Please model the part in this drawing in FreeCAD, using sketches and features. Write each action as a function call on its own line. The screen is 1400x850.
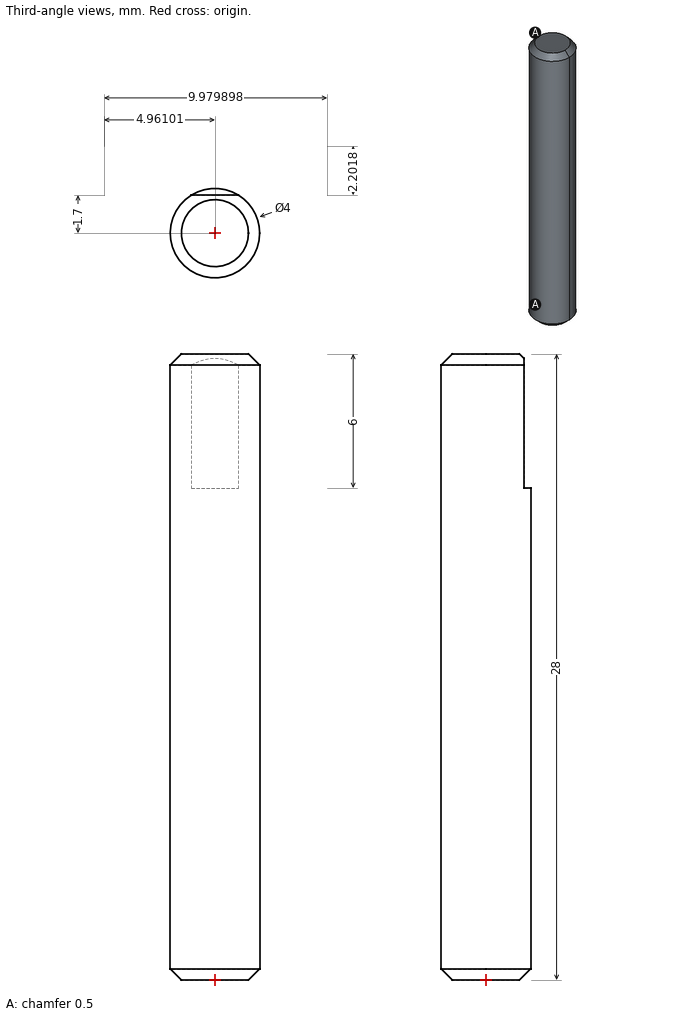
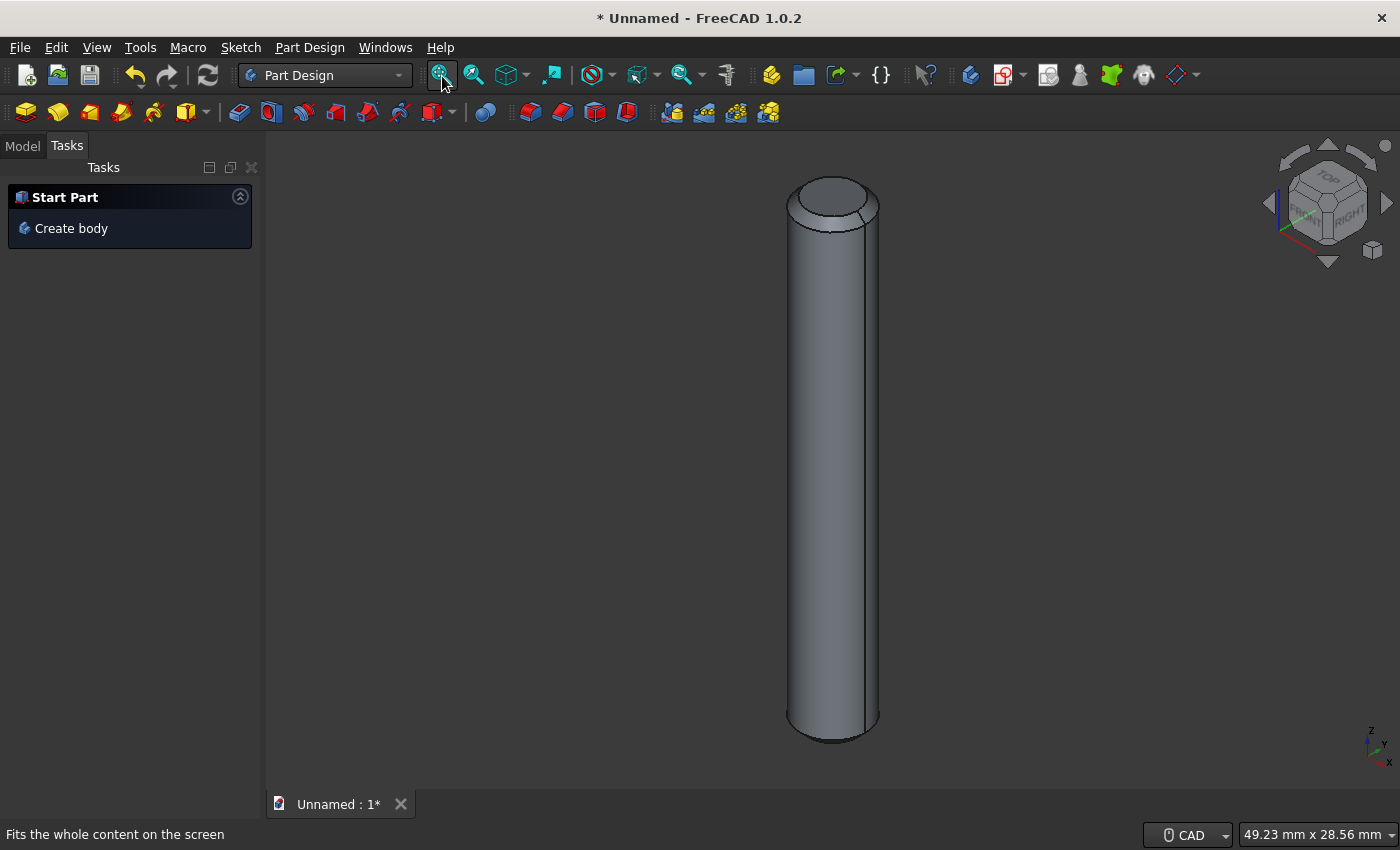
click(833, 196)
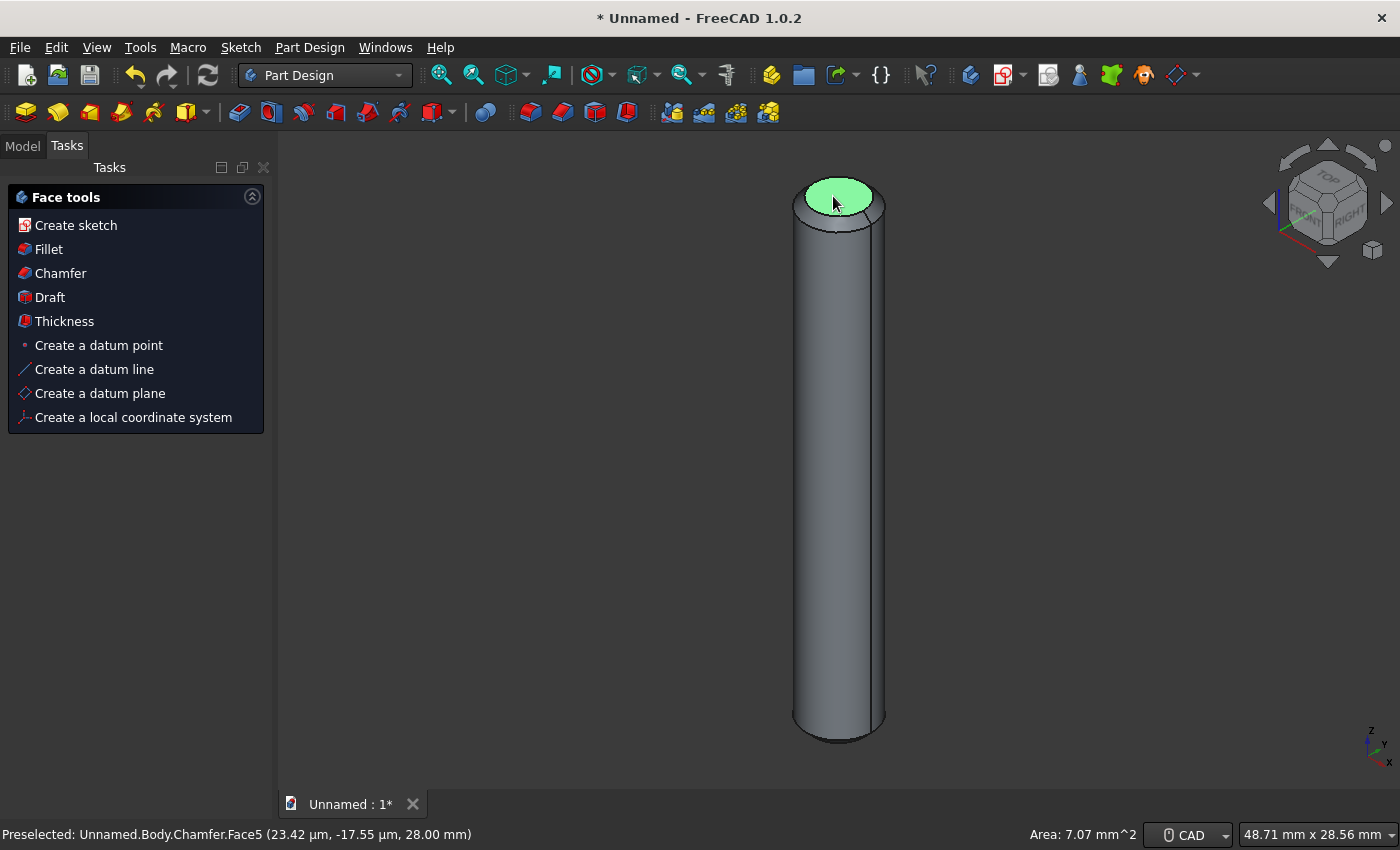
click(1004, 76)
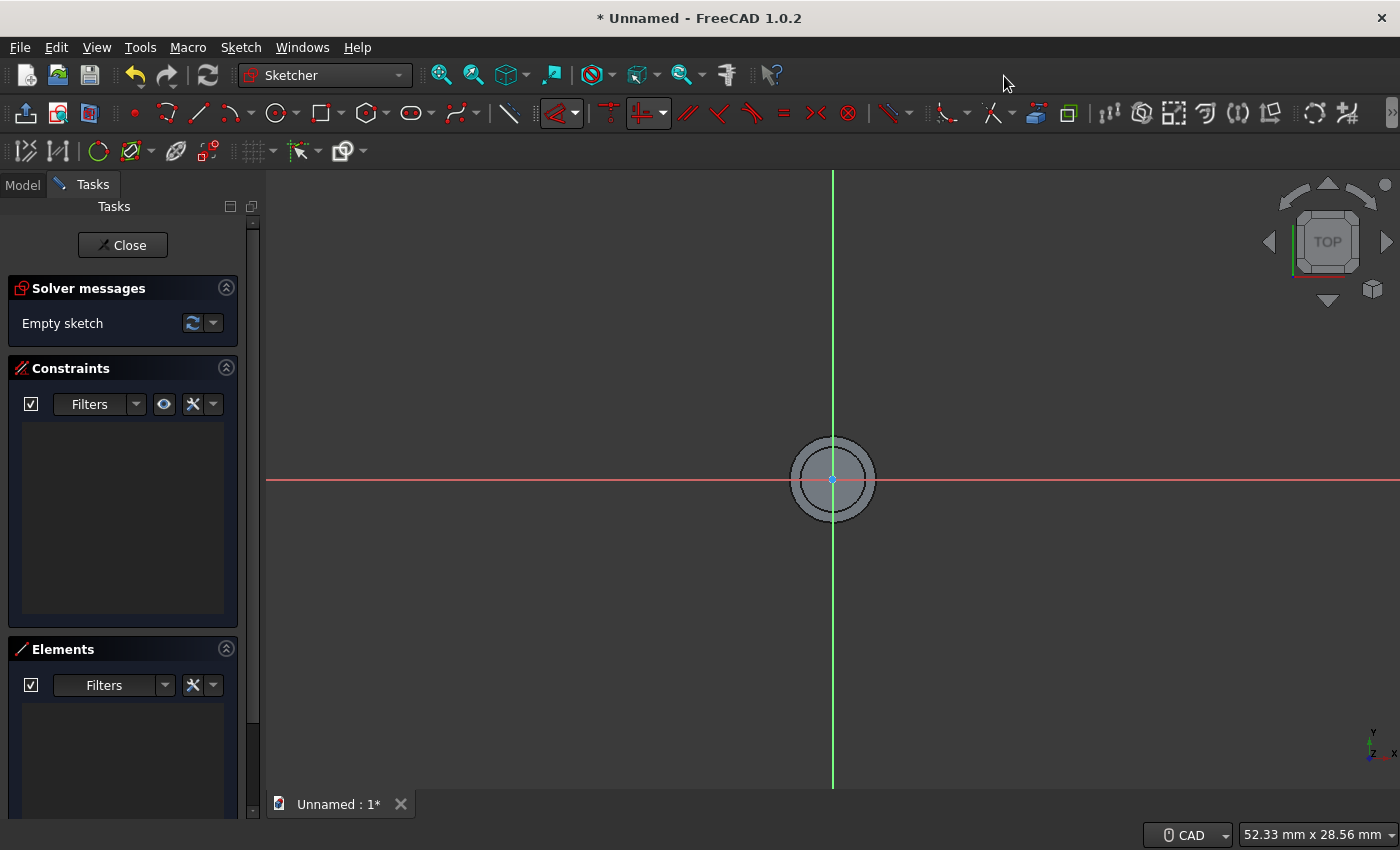
scroll(863, 419, up, 6)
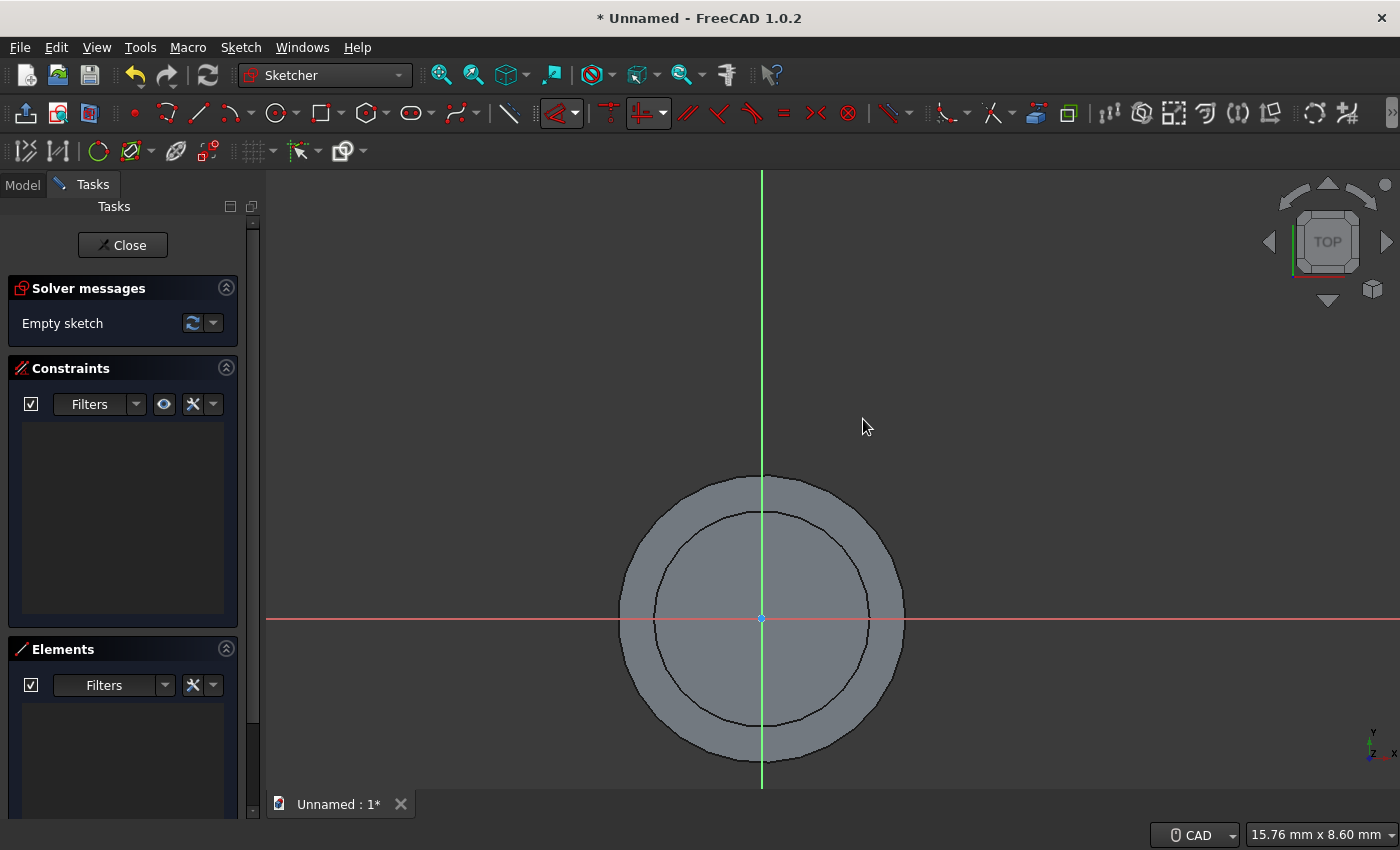
click(322, 114)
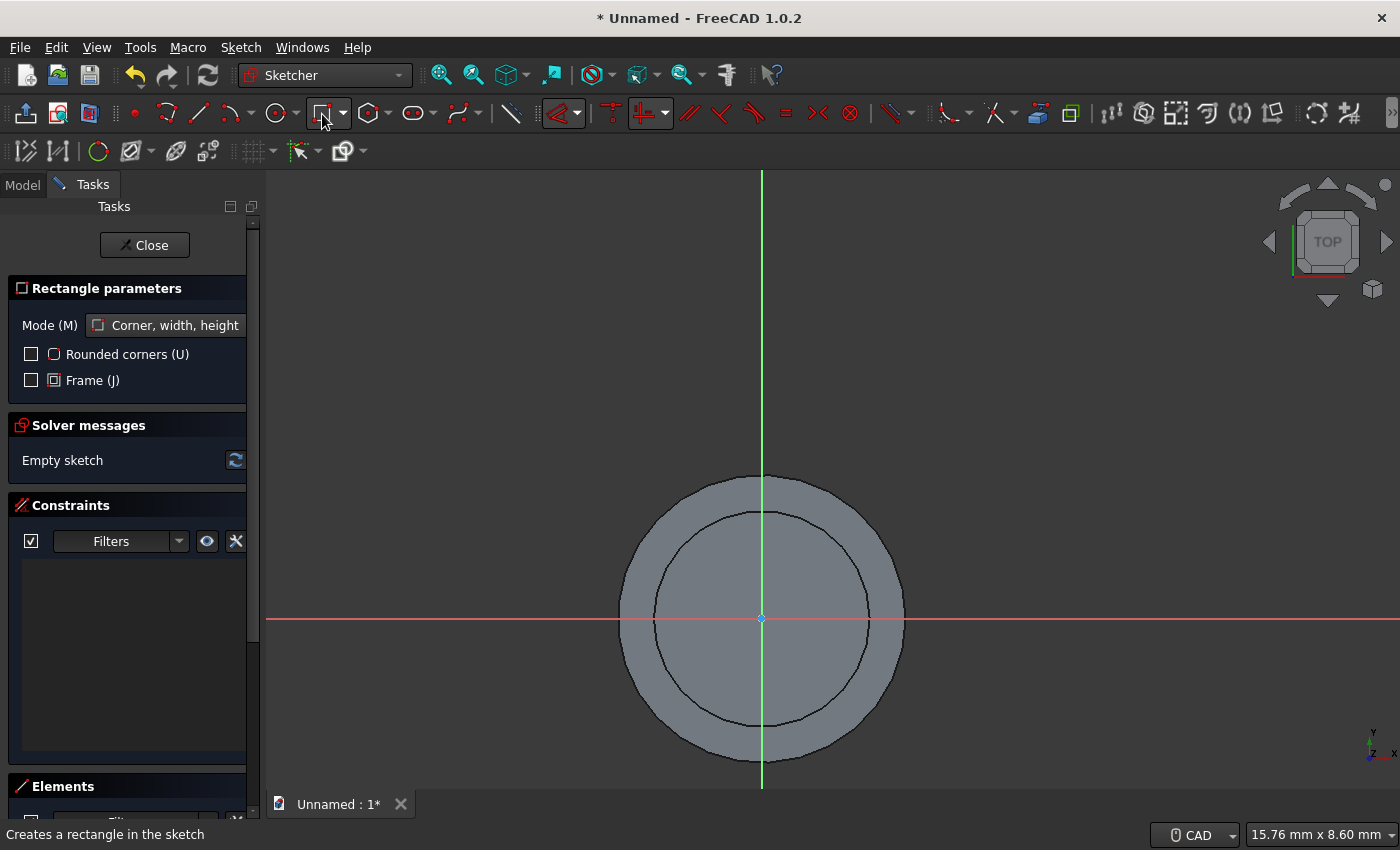
click(405, 338)
move(1123, 497)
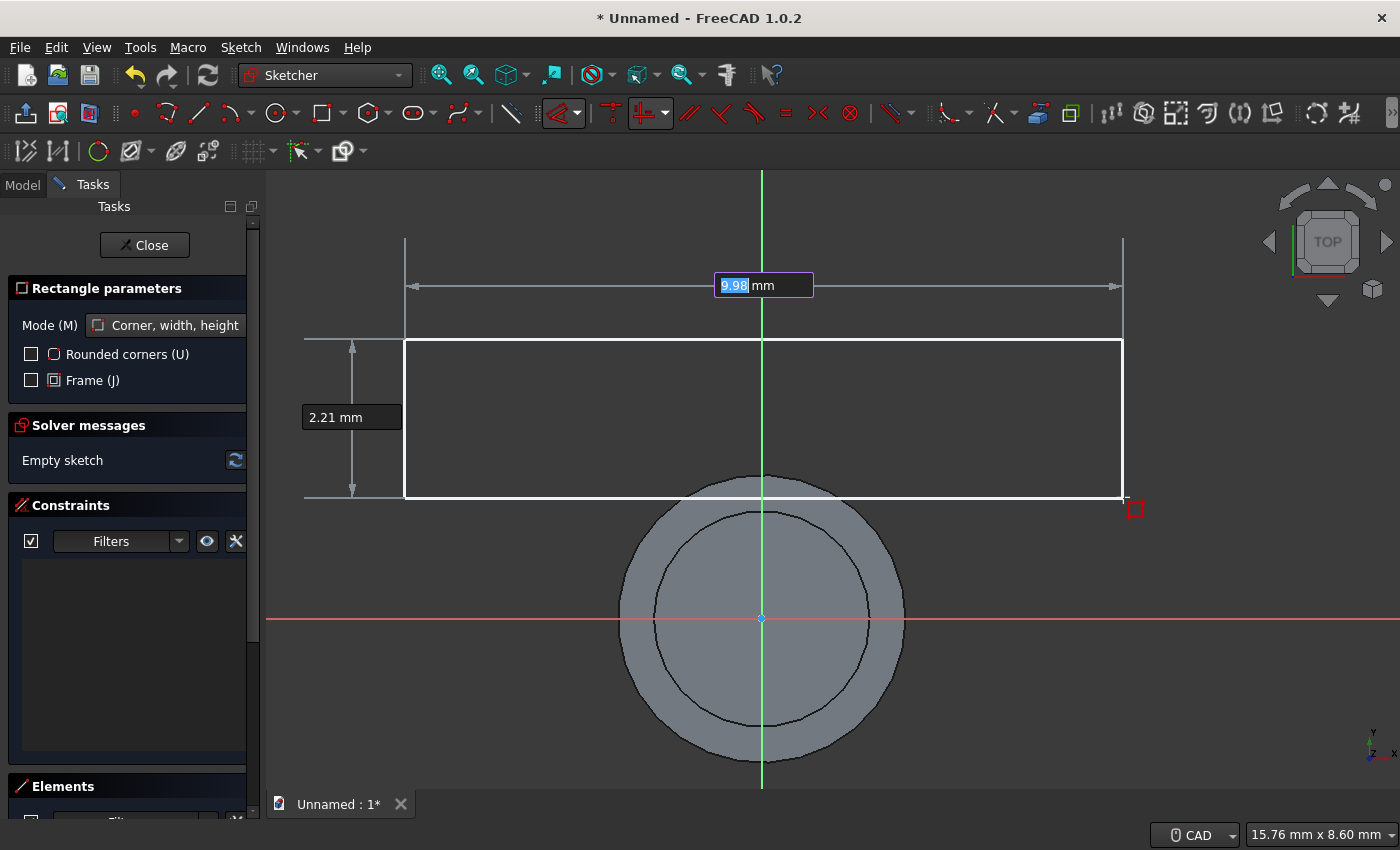
text(9.979898)
key(Tab)
text(2.2018)
key(Return)
key(Escape)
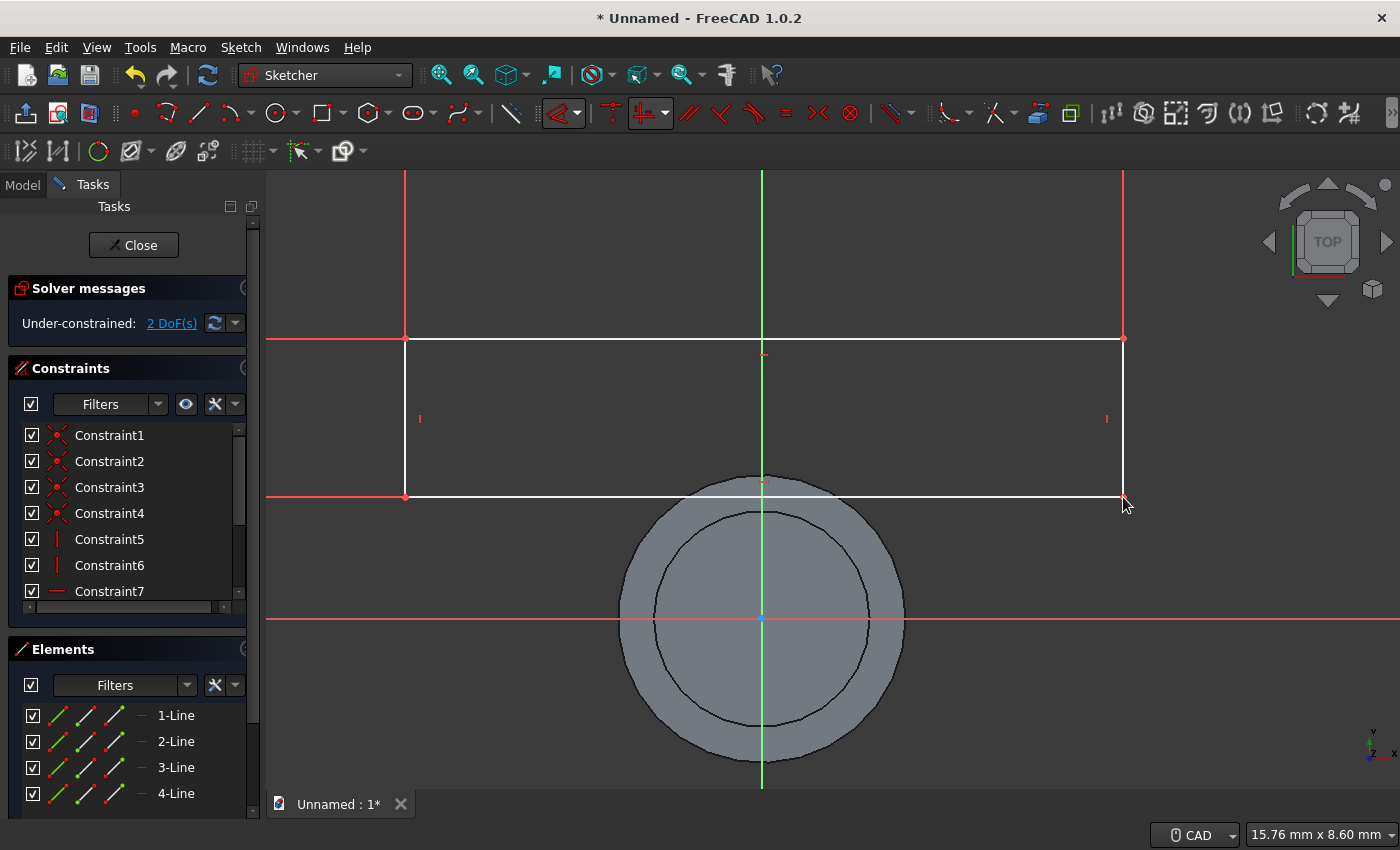
click(558, 114)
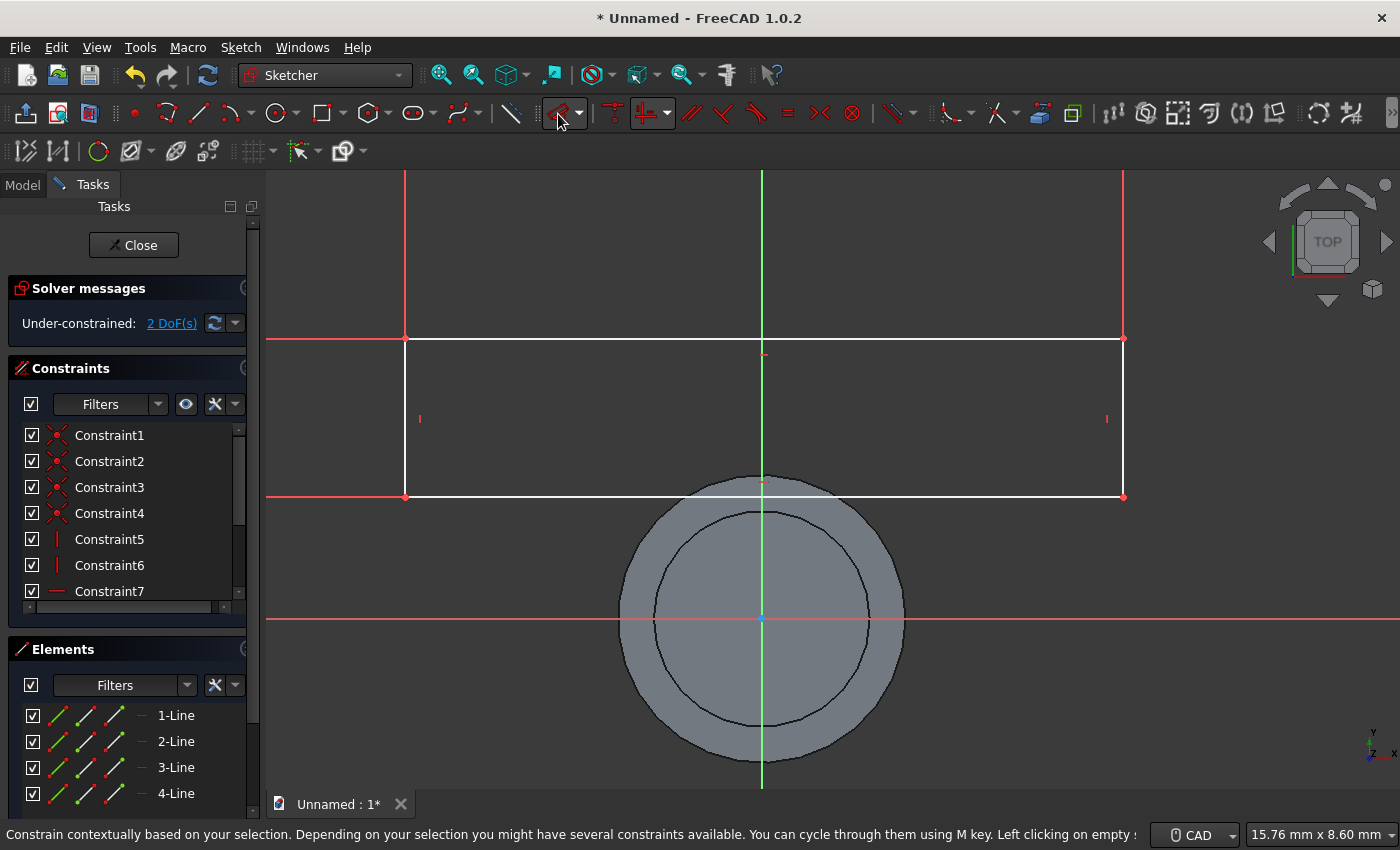
click(405, 497)
click(371, 558)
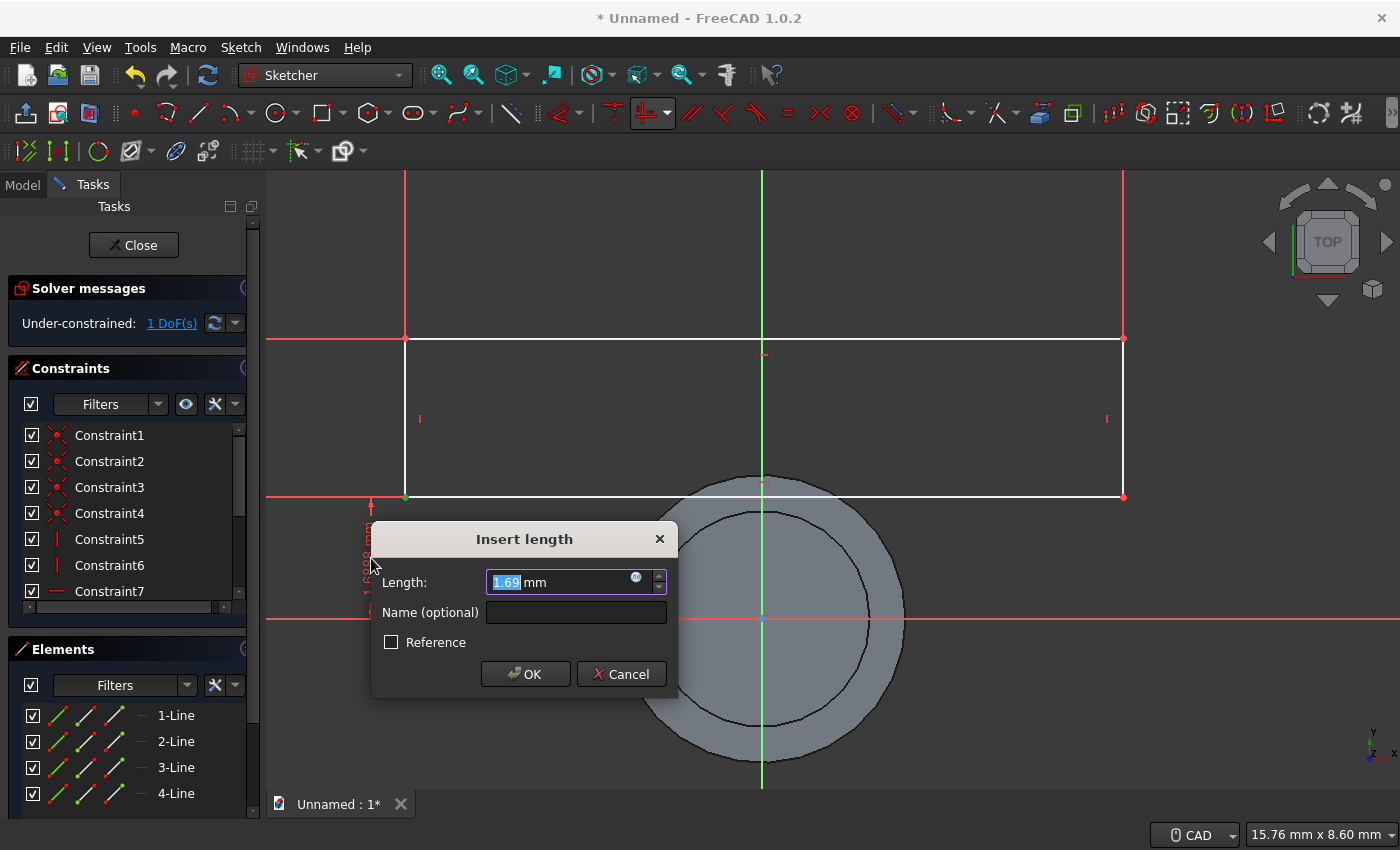
text(1.7)
key(Return)